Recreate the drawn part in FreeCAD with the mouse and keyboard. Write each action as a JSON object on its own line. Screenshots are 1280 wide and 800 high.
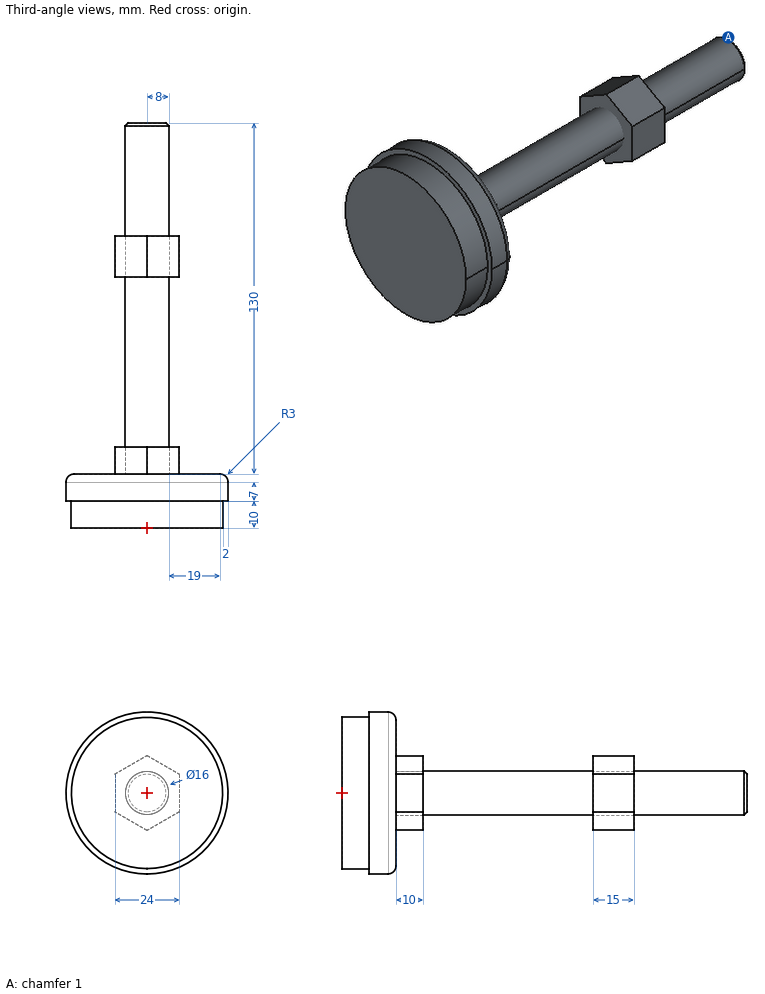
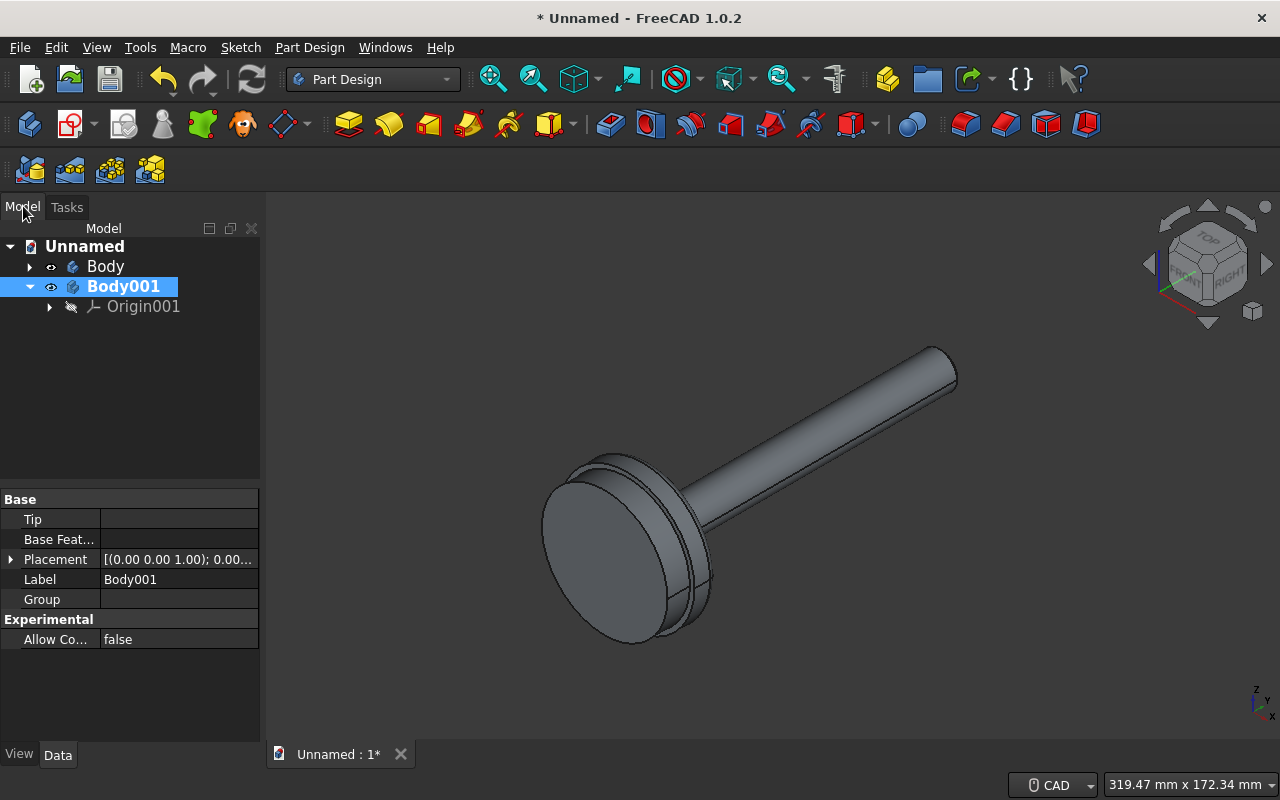
{"action": "left_click", "coordinate": [50, 307]}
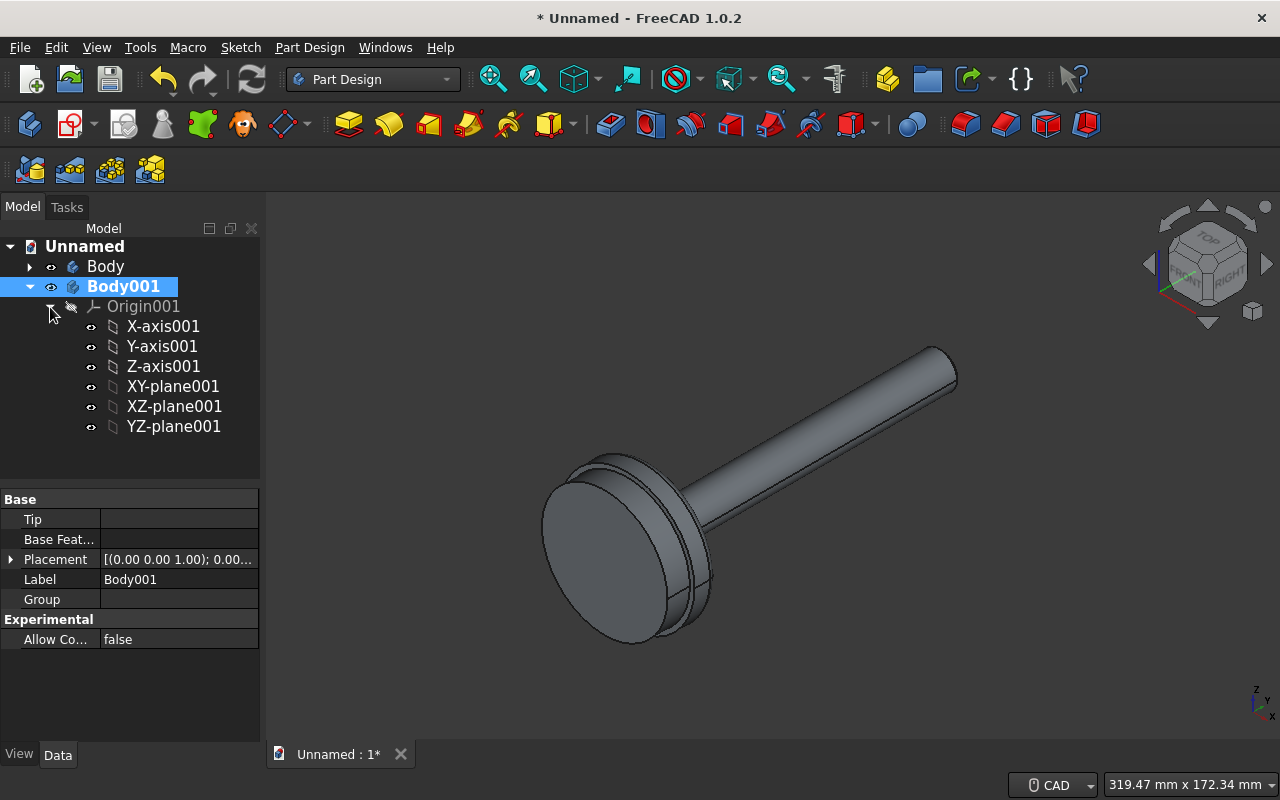
{"action": "left_click", "coordinate": [136, 407]}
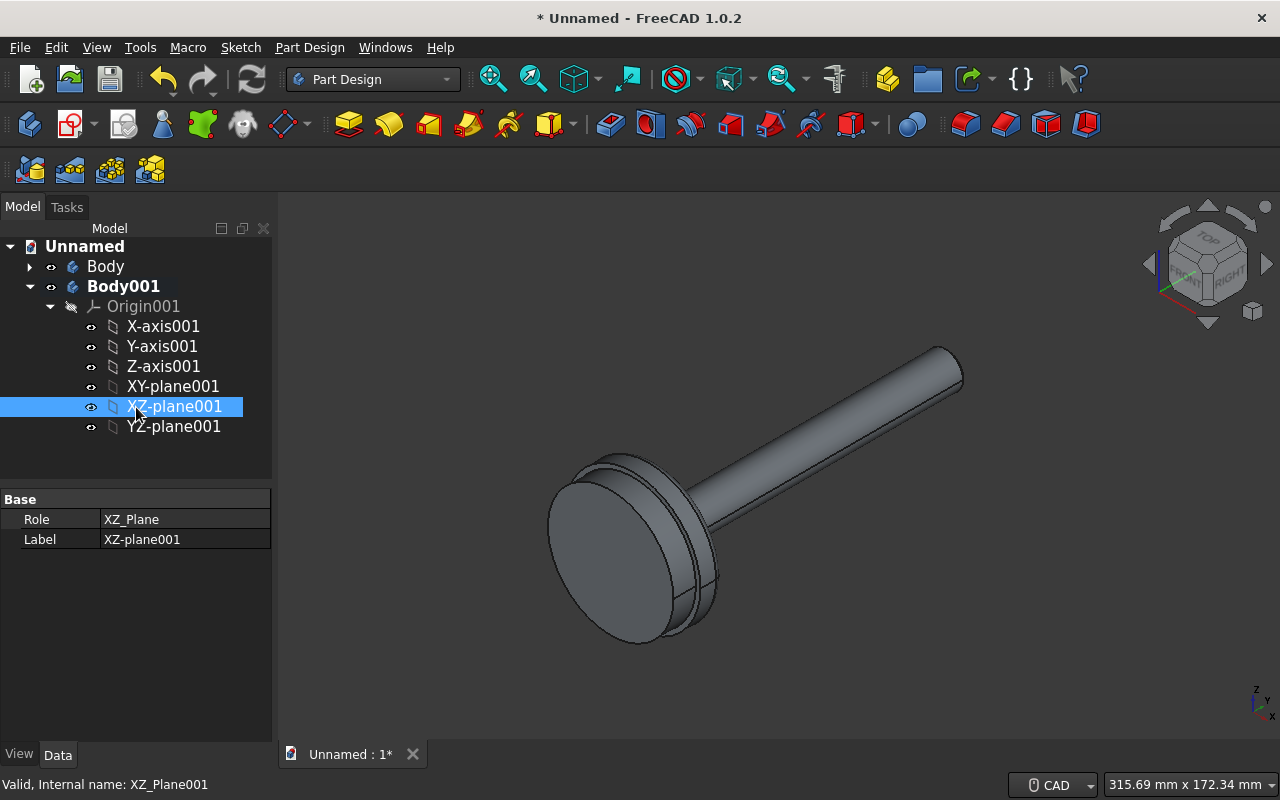
{"action": "left_click", "coordinate": [284, 124]}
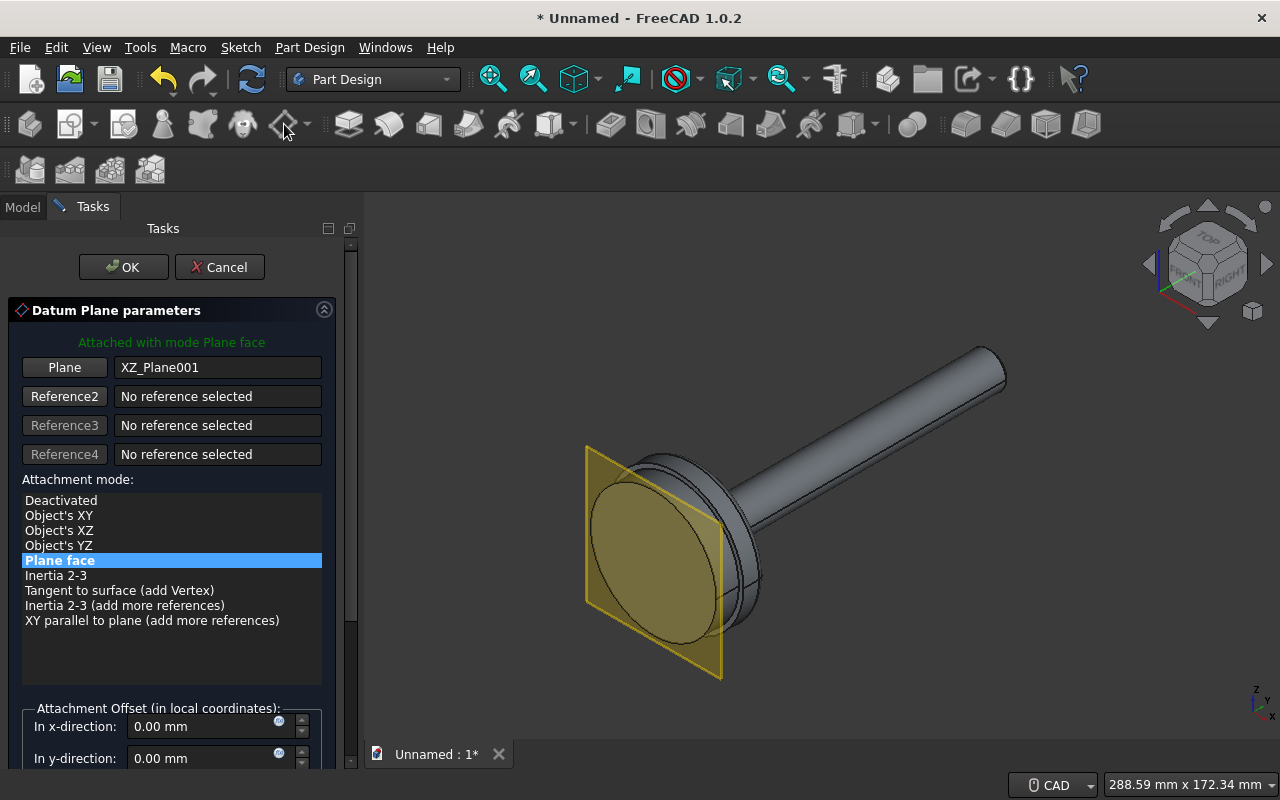
{"action": "scroll", "coordinate": [351, 503], "scroll_direction": "down", "scroll_amount": 2}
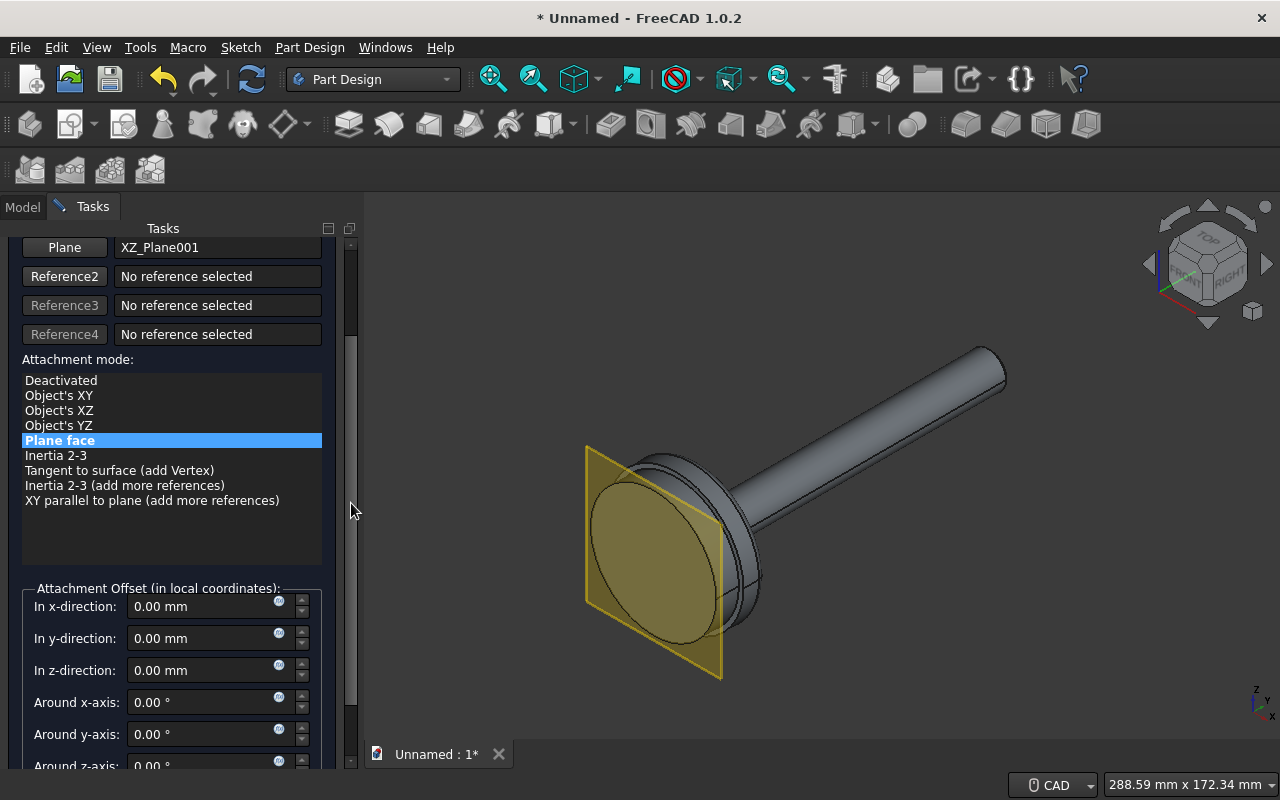
{"action": "triple_click", "coordinate": [210, 670]}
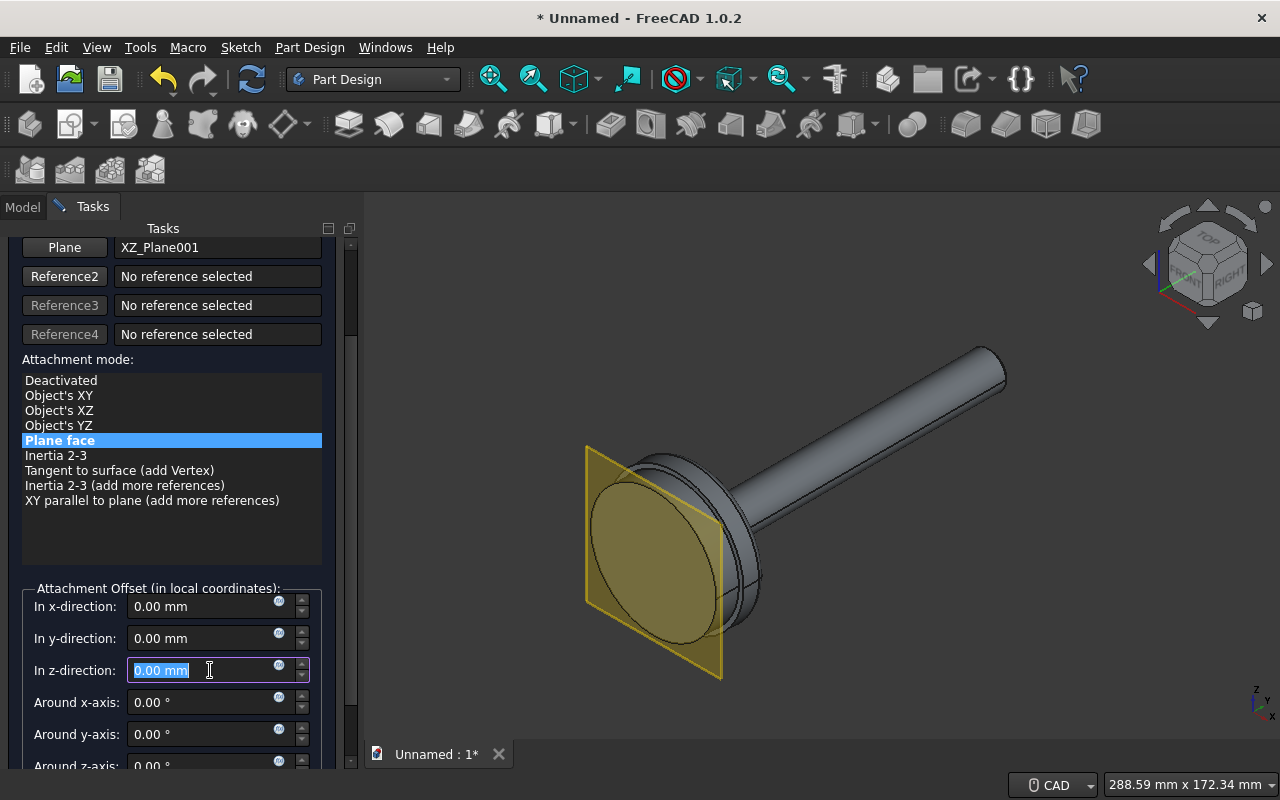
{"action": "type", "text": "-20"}
{"action": "key", "text": "Tab"}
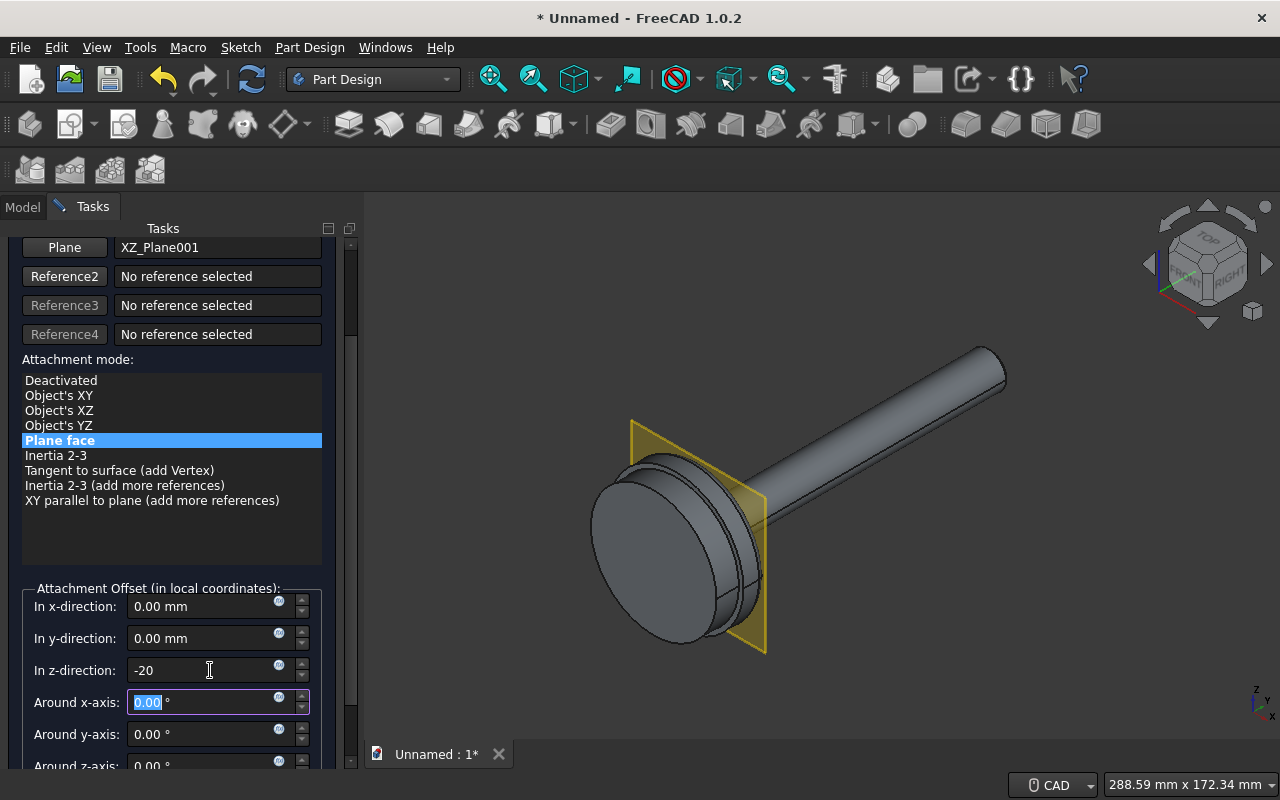
{"action": "scroll", "coordinate": [351, 503], "scroll_direction": "up", "scroll_amount": 3}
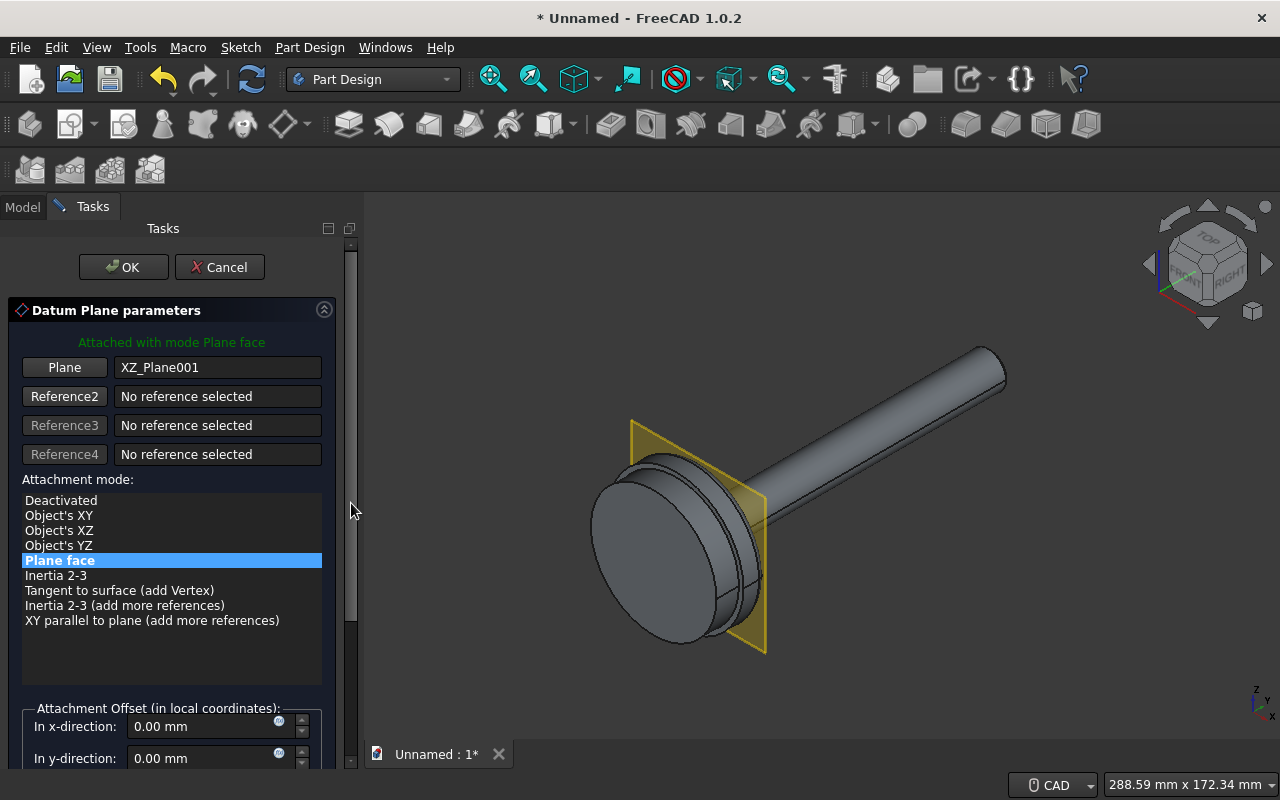
{"action": "left_click", "coordinate": [124, 267]}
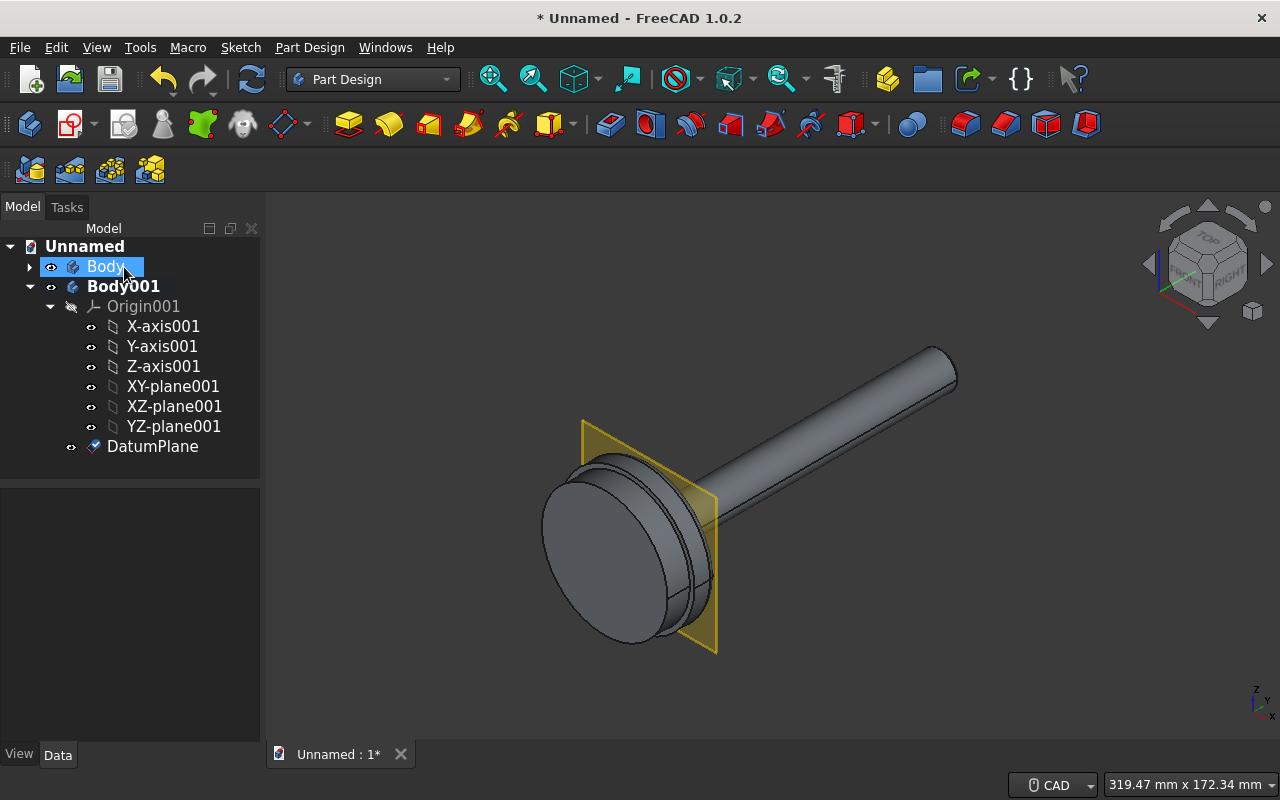
{"action": "left_click", "coordinate": [116, 447]}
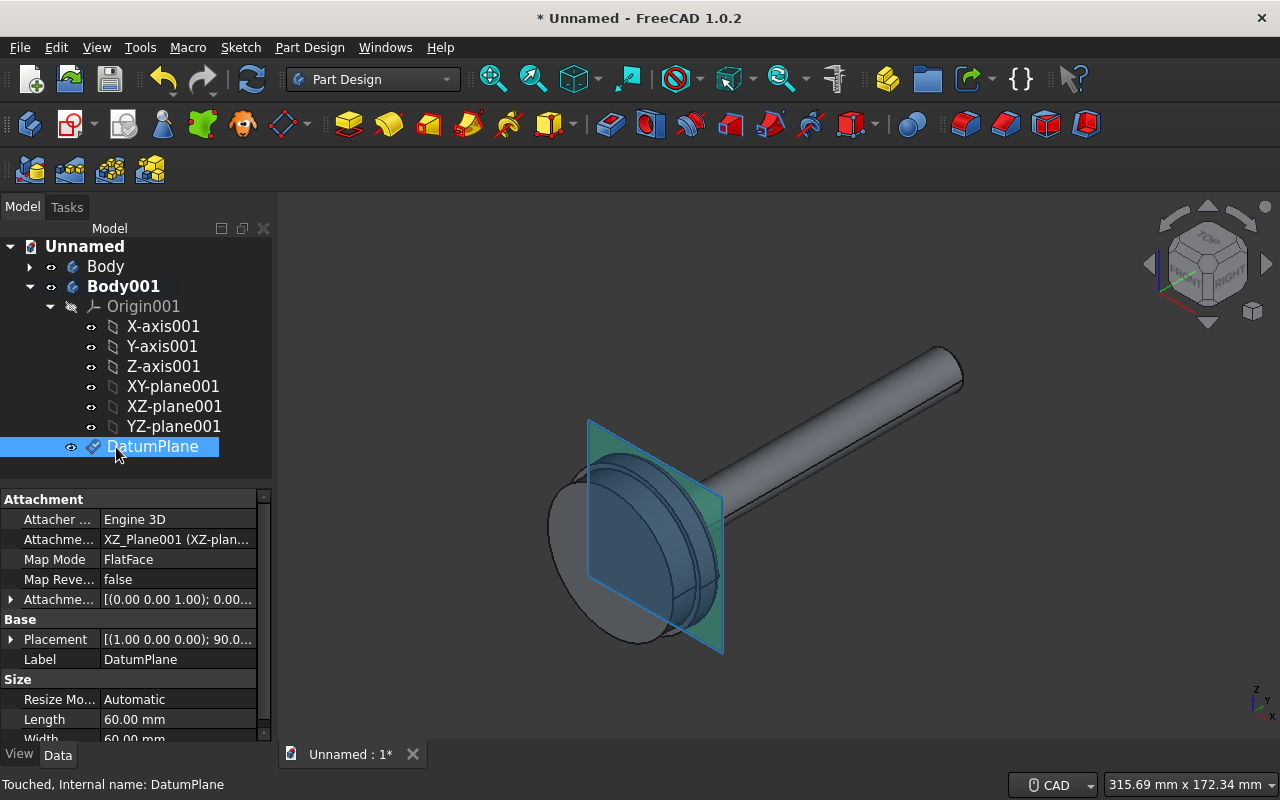
{"action": "left_click", "coordinate": [70, 124]}